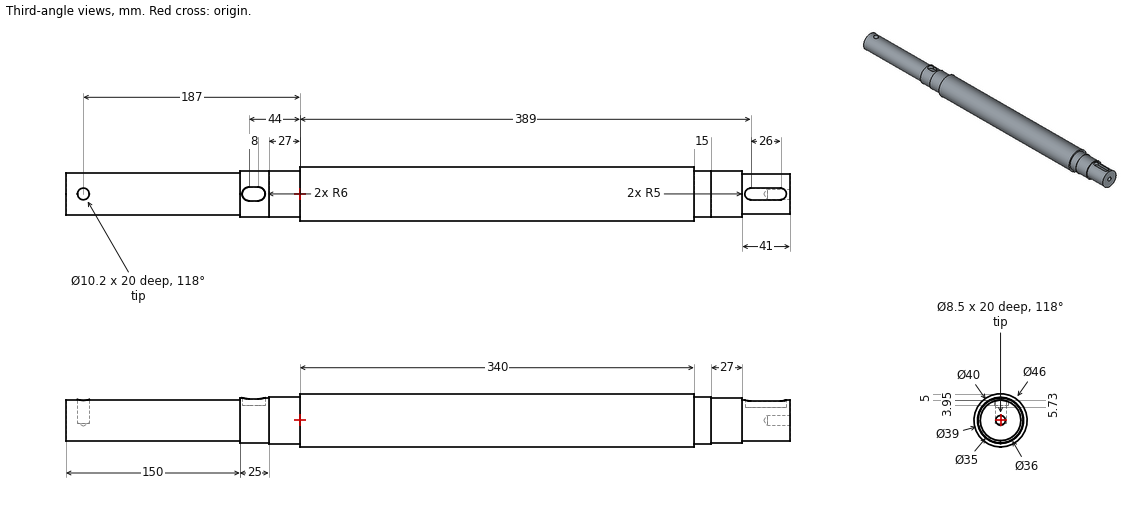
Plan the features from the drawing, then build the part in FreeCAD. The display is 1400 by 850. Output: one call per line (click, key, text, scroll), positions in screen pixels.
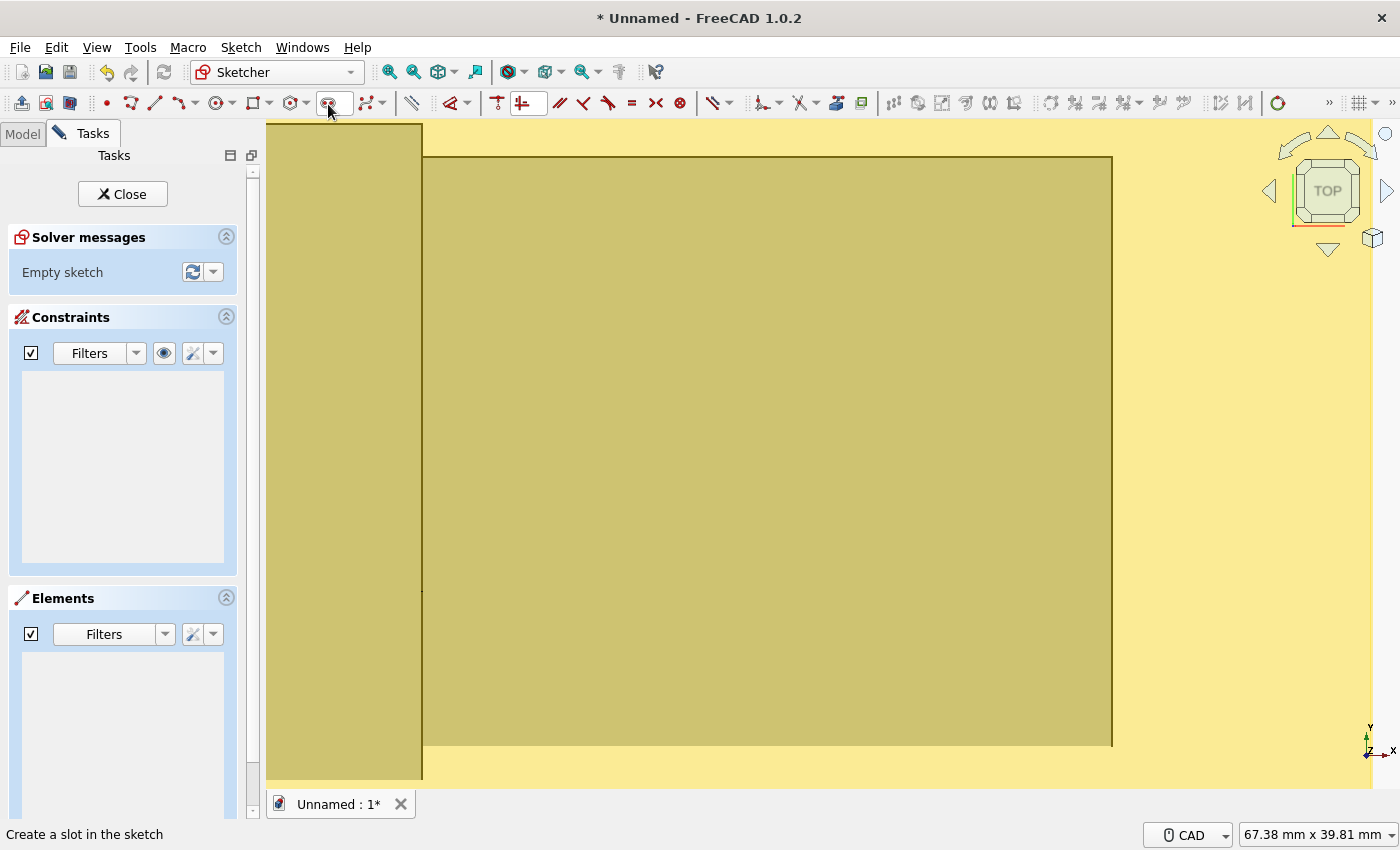
click(539, 452)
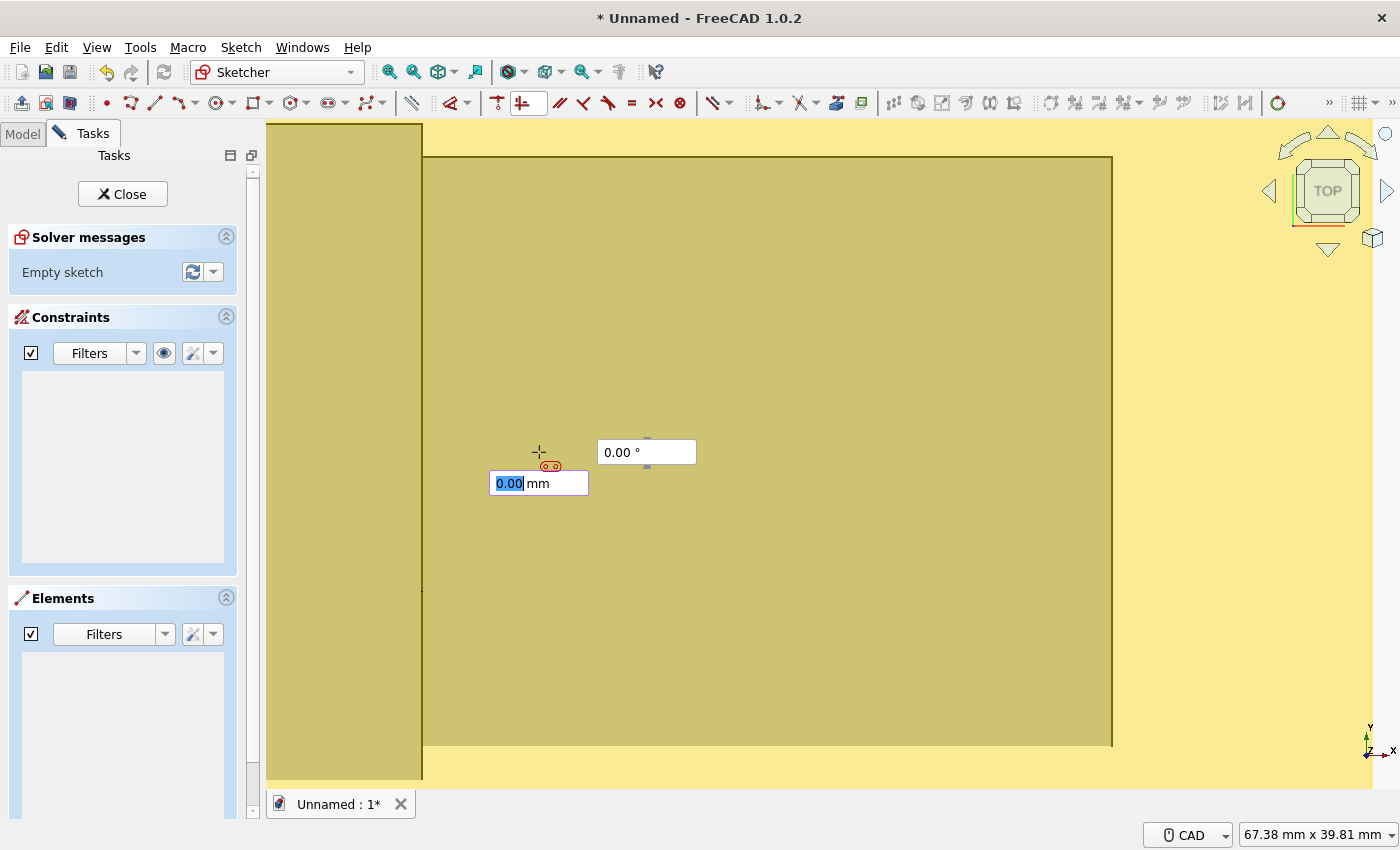
click(977, 443)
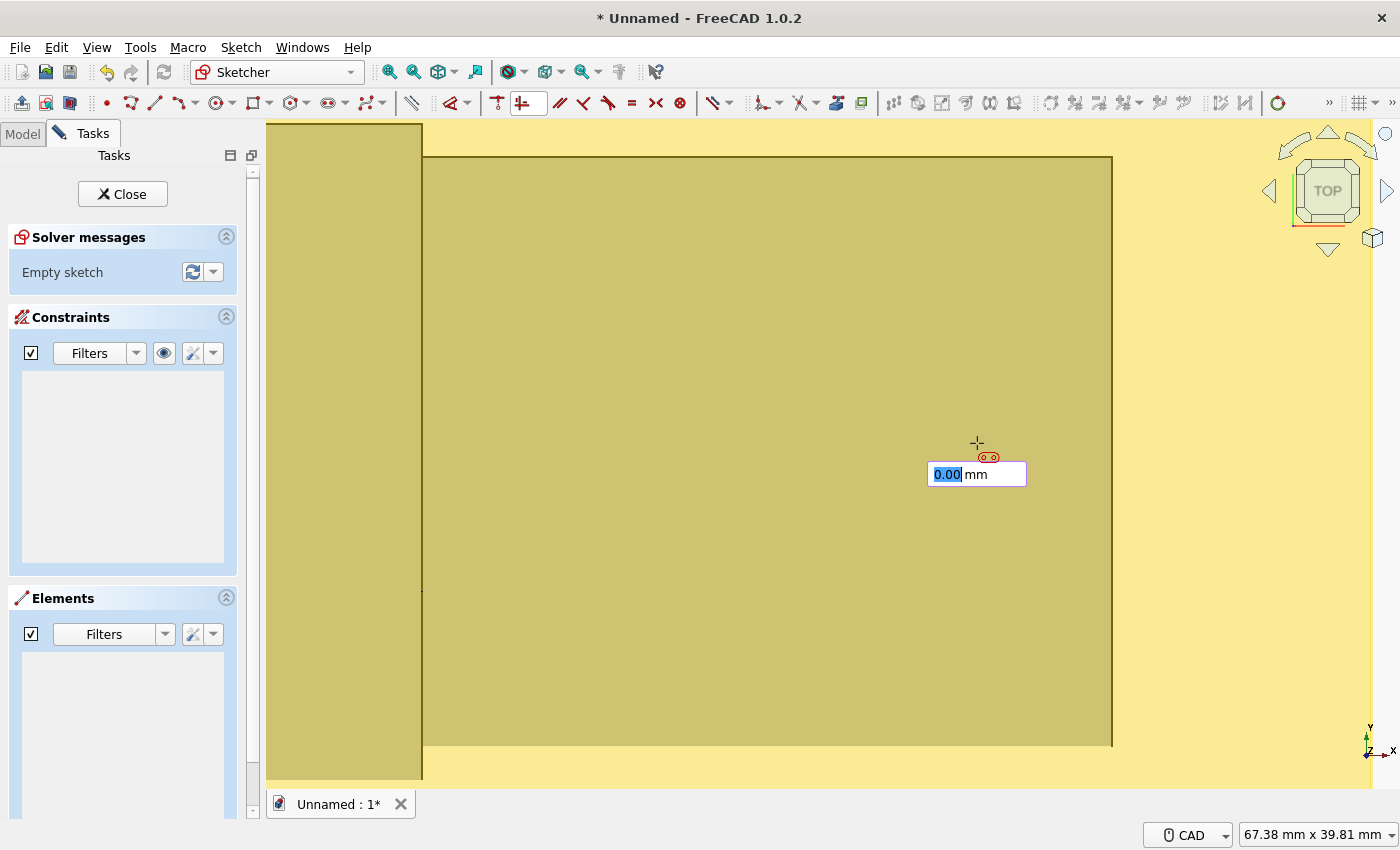
click(758, 368)
key(Escape)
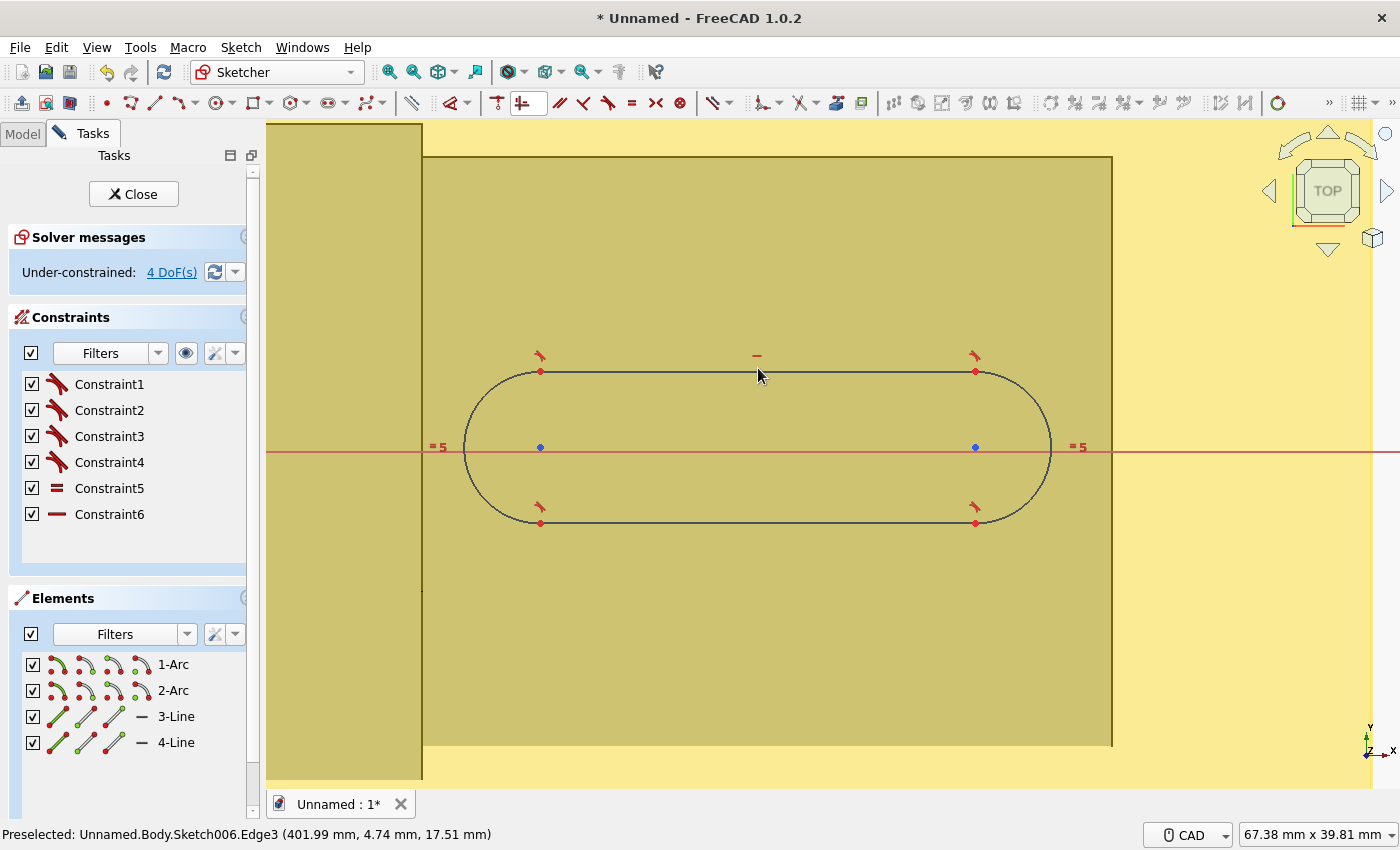
click(540, 448)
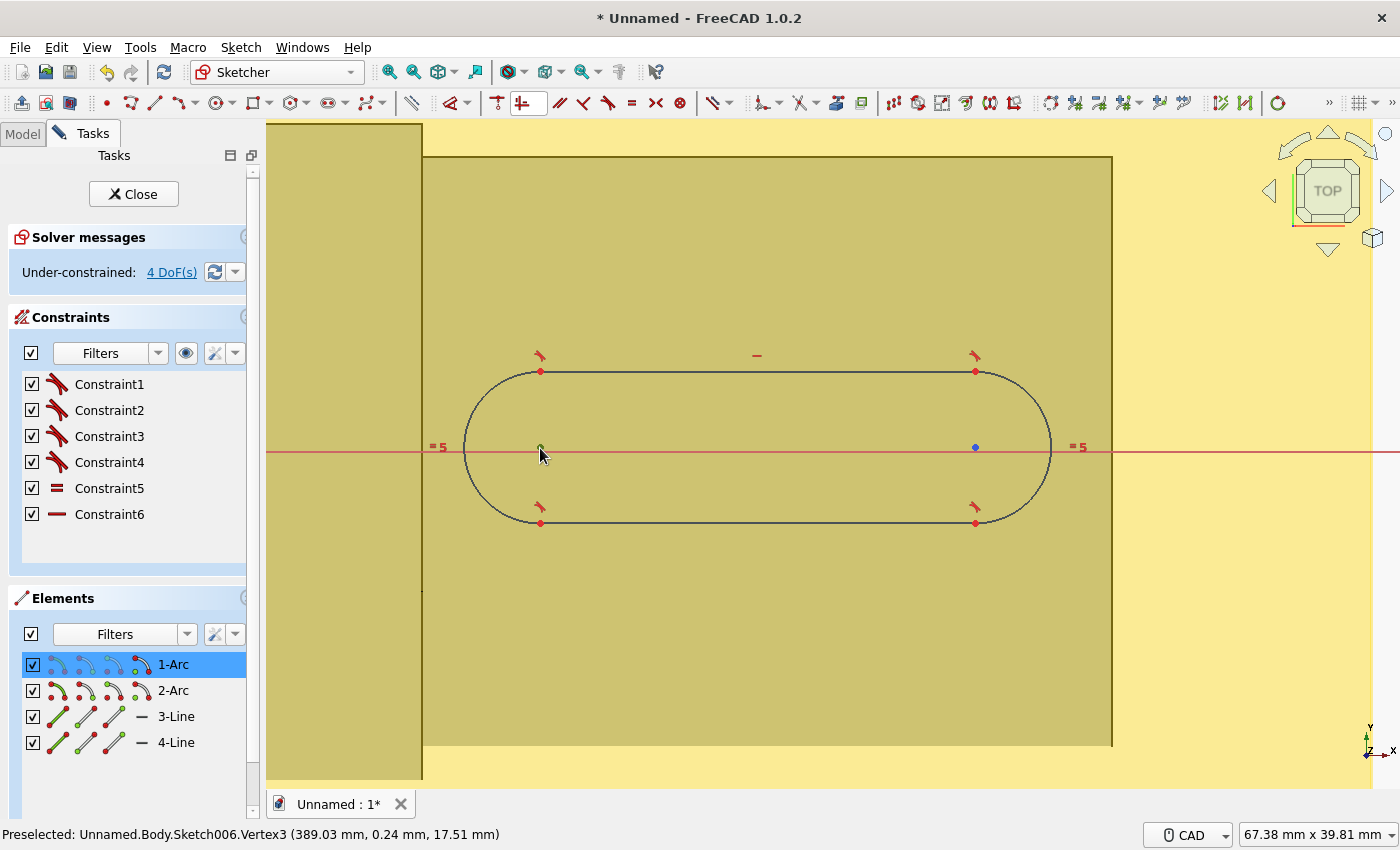
click(361, 452)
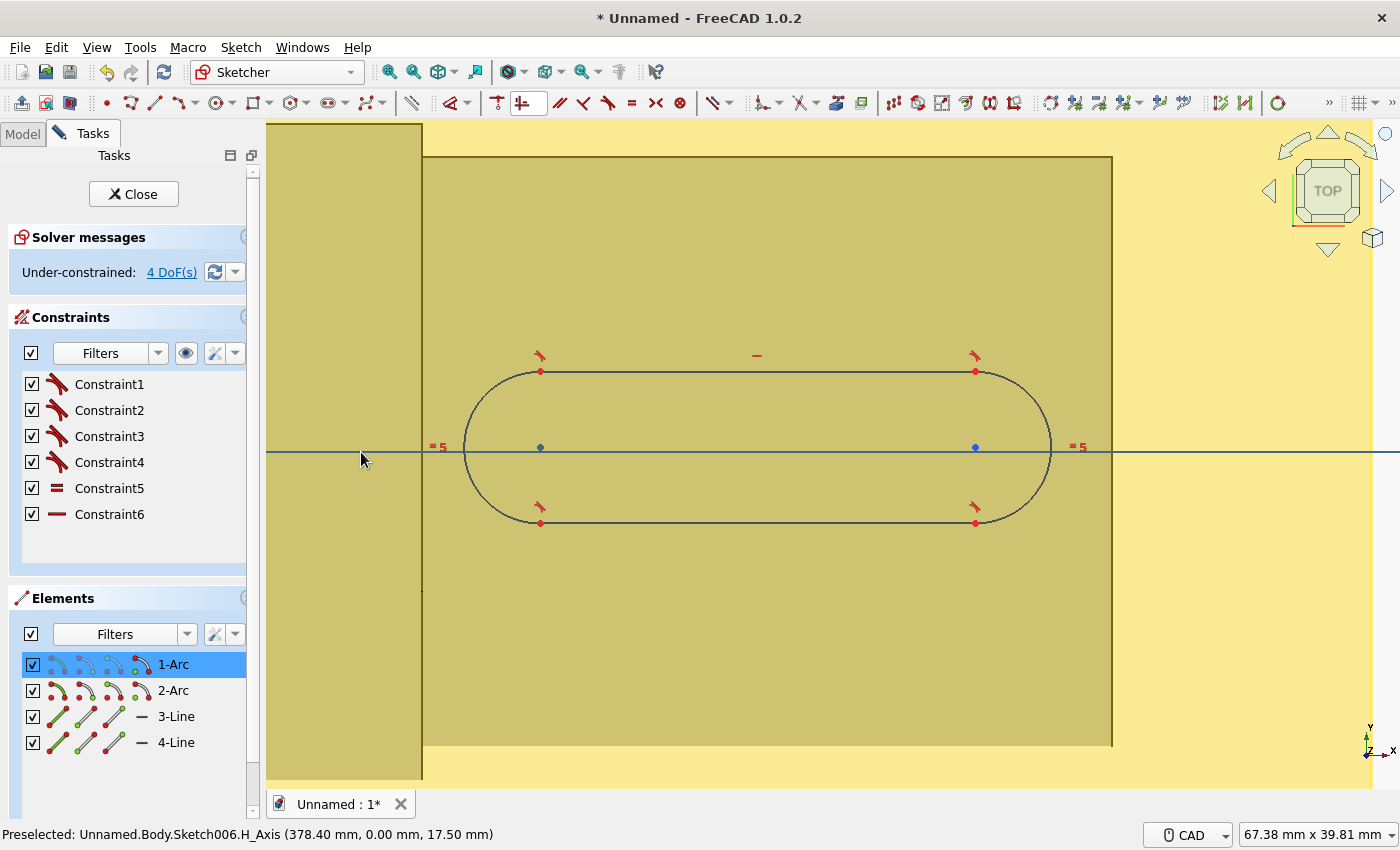
click(498, 104)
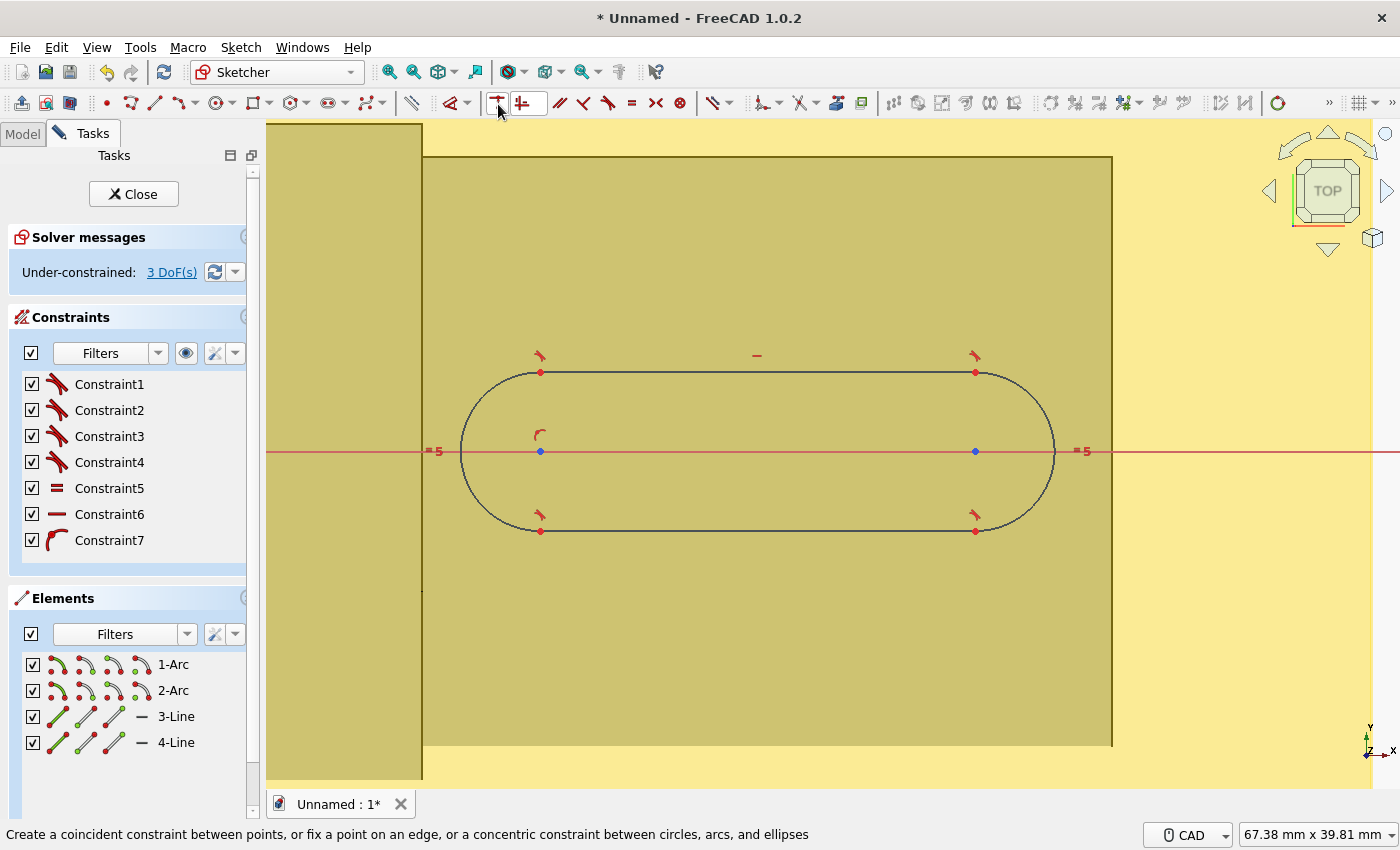
click(450, 104)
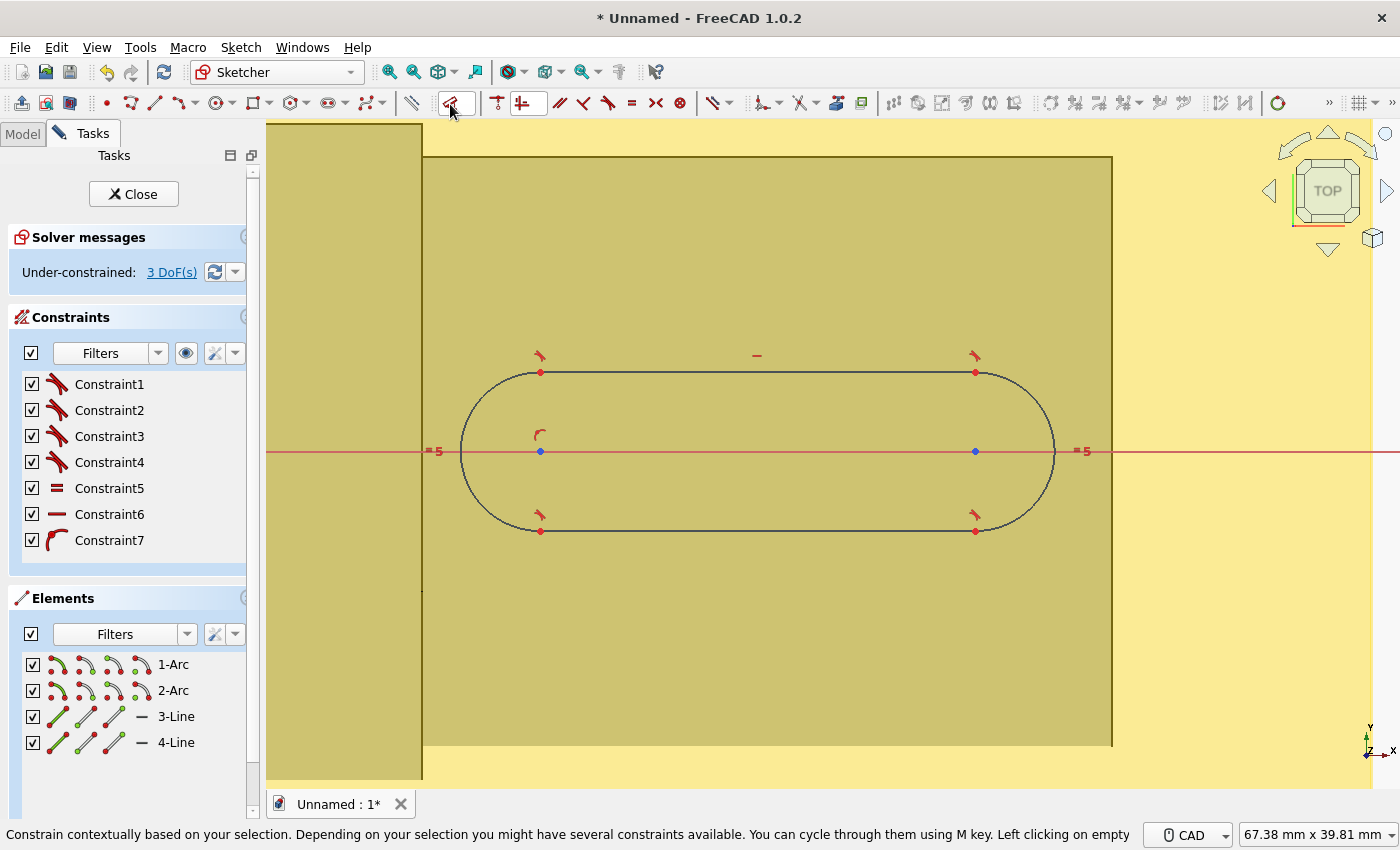
click(476, 405)
click(450, 386)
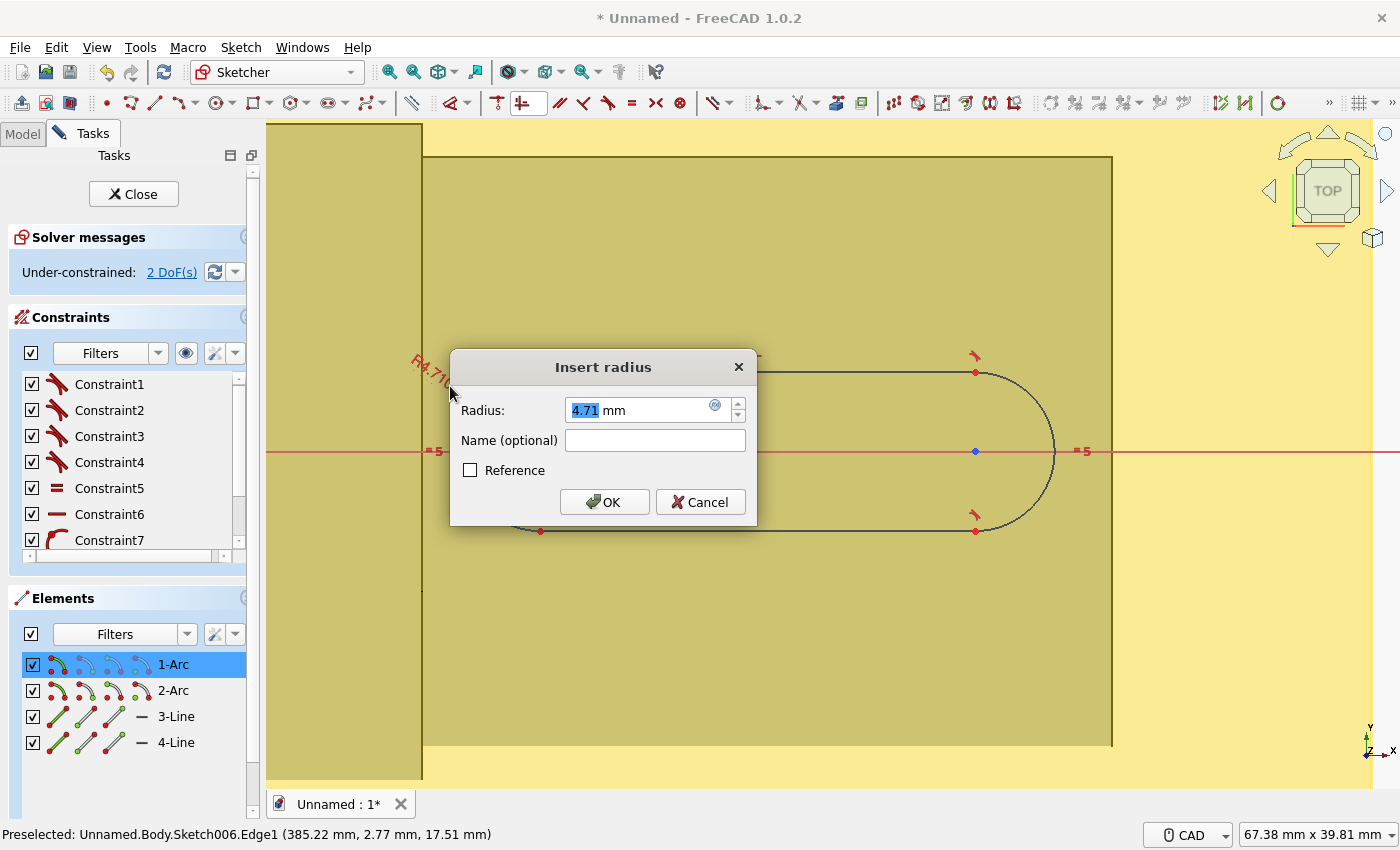
text(5)
key(Return)